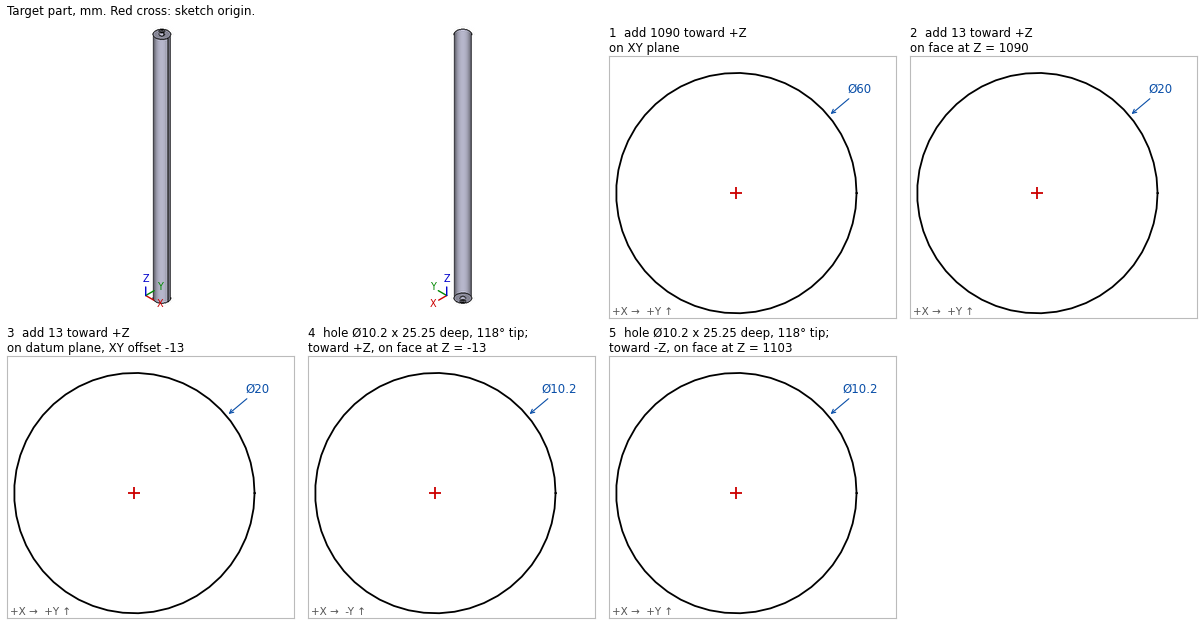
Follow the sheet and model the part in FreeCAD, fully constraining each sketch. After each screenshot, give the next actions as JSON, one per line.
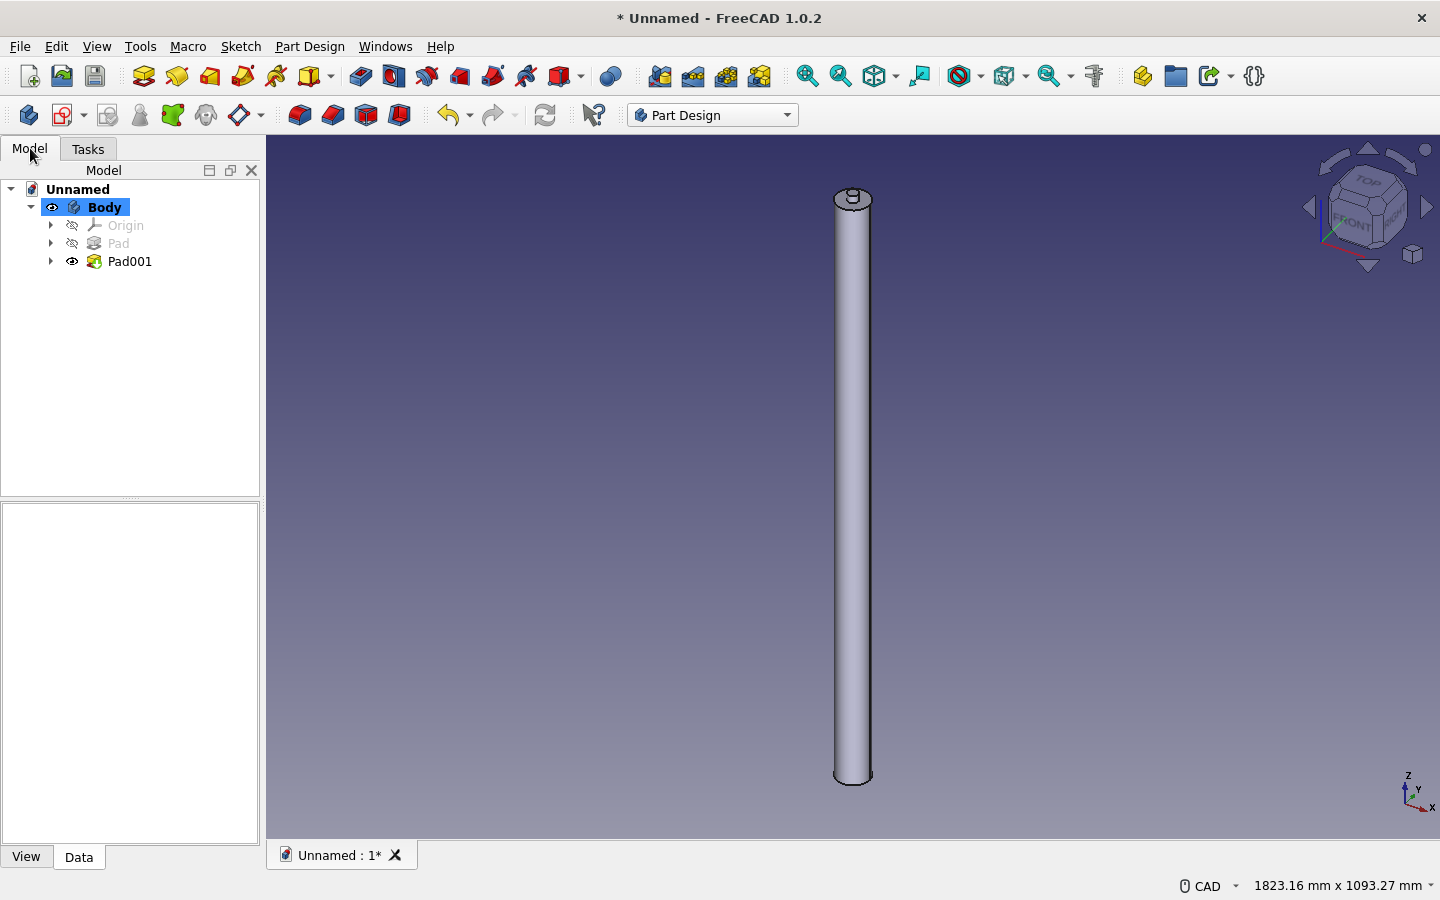
{"action": "left_click", "coordinate": [51, 225]}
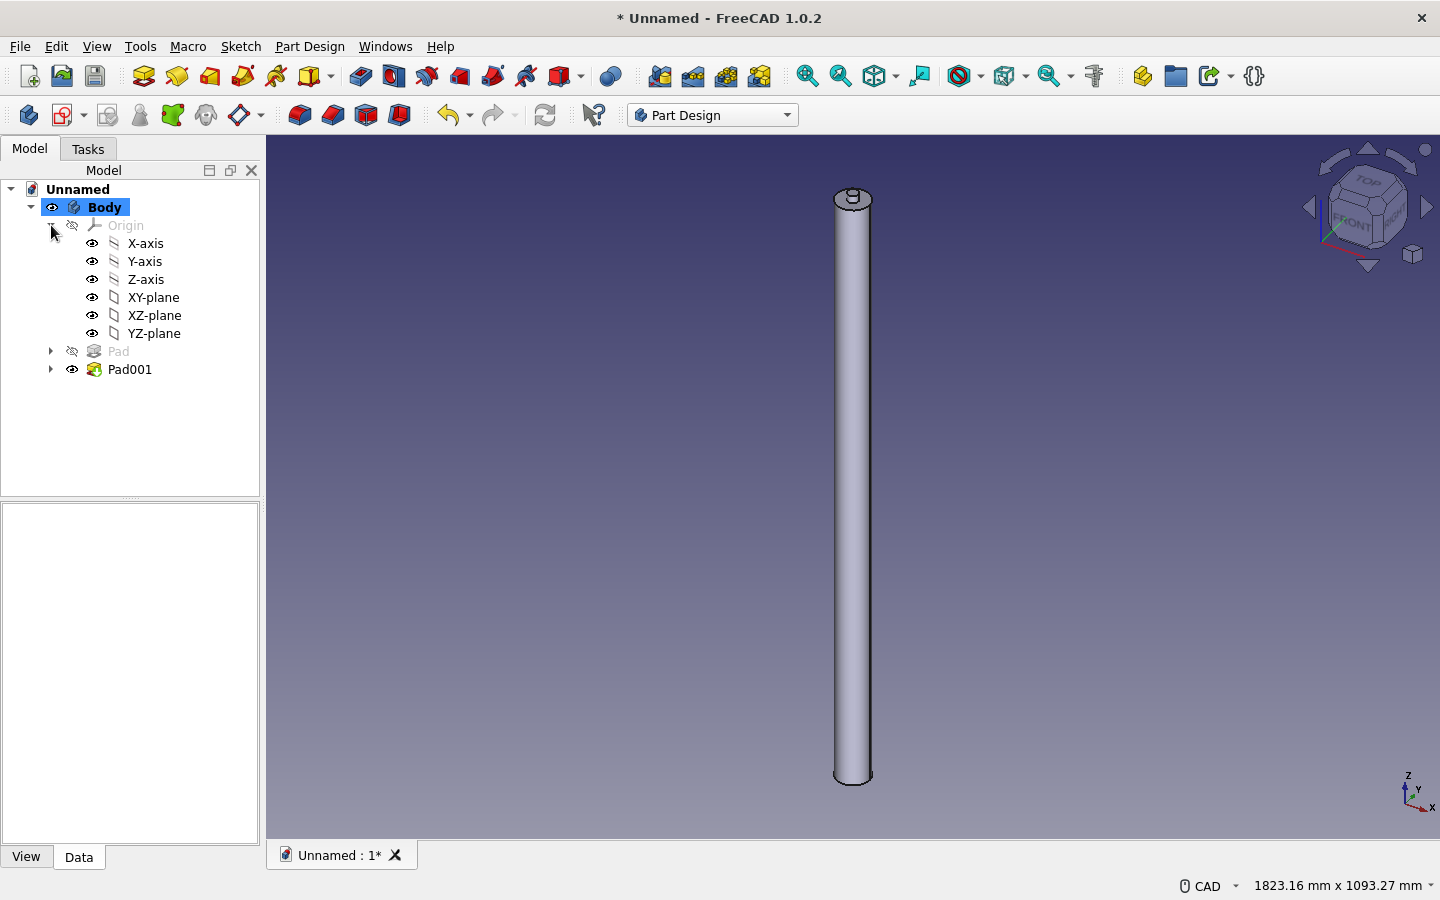
{"action": "left_click", "coordinate": [137, 297]}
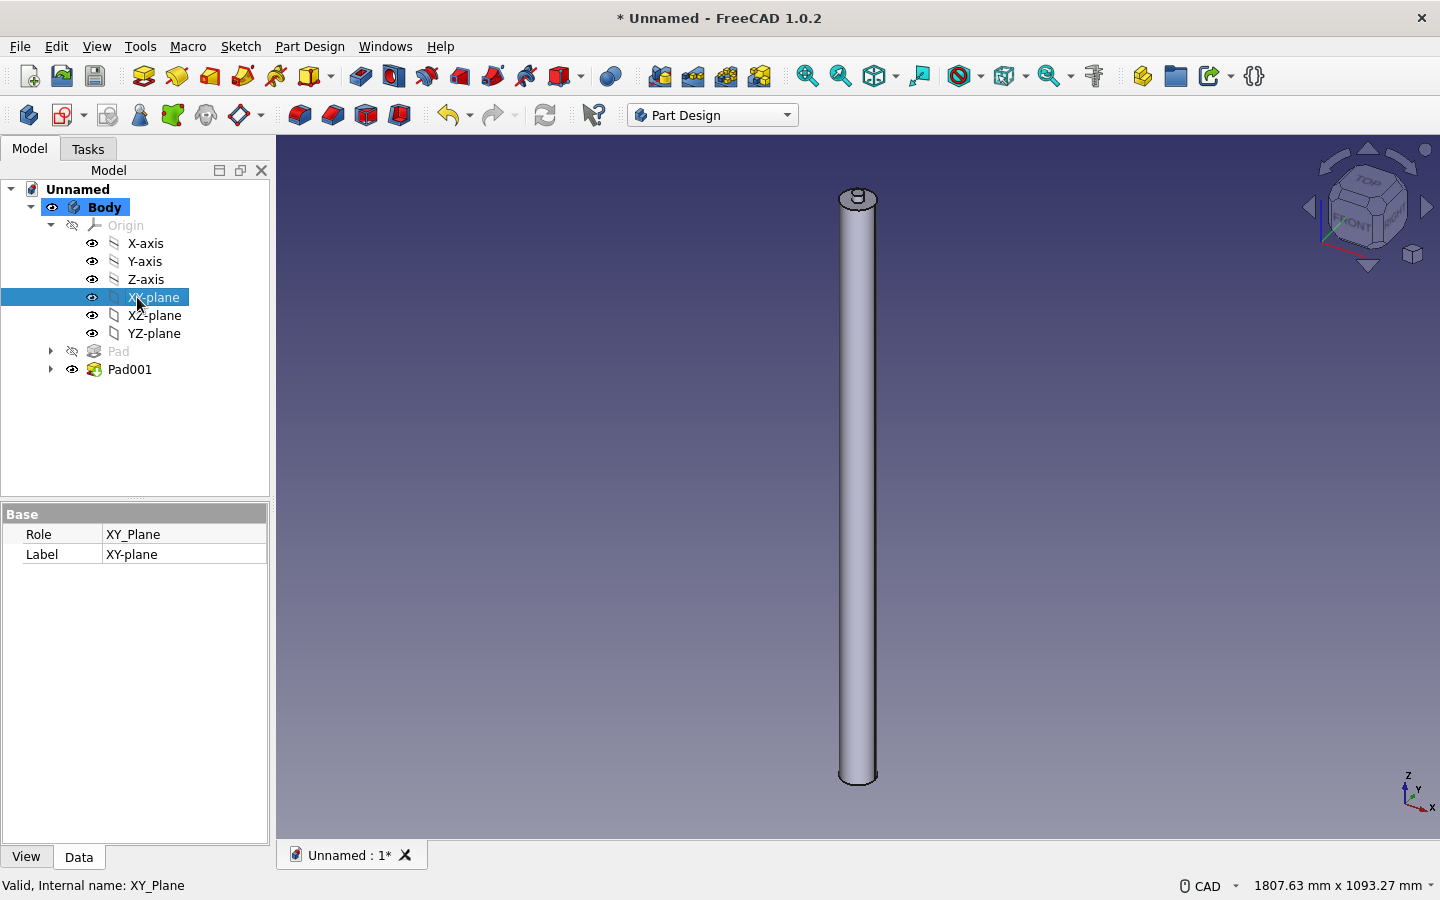
{"action": "left_click", "coordinate": [238, 116]}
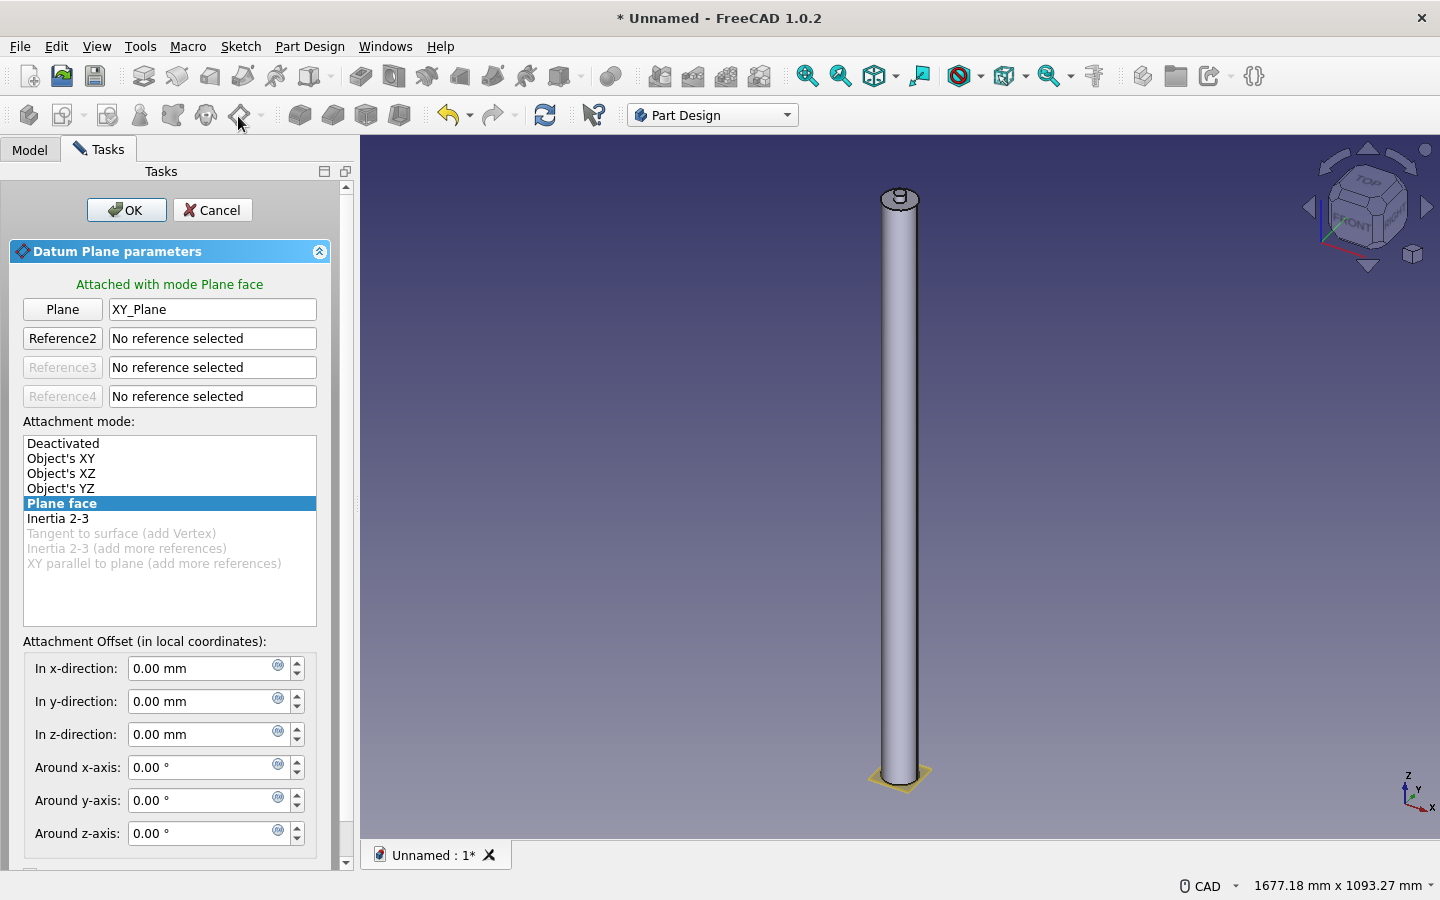
{"action": "triple_click", "coordinate": [210, 734]}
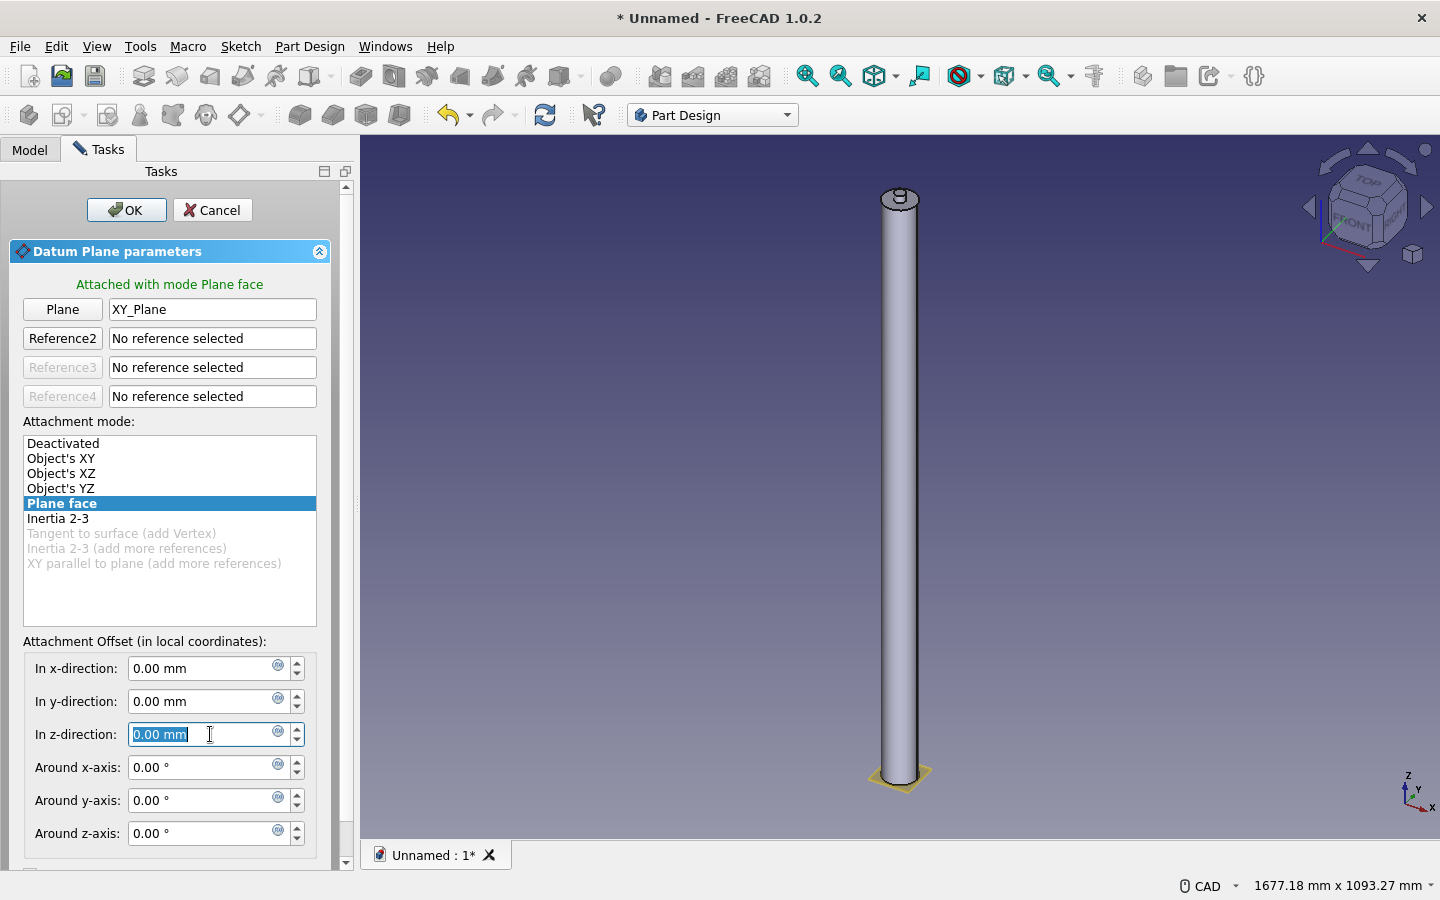
{"action": "type", "text": "-13"}
{"action": "key", "text": "Tab"}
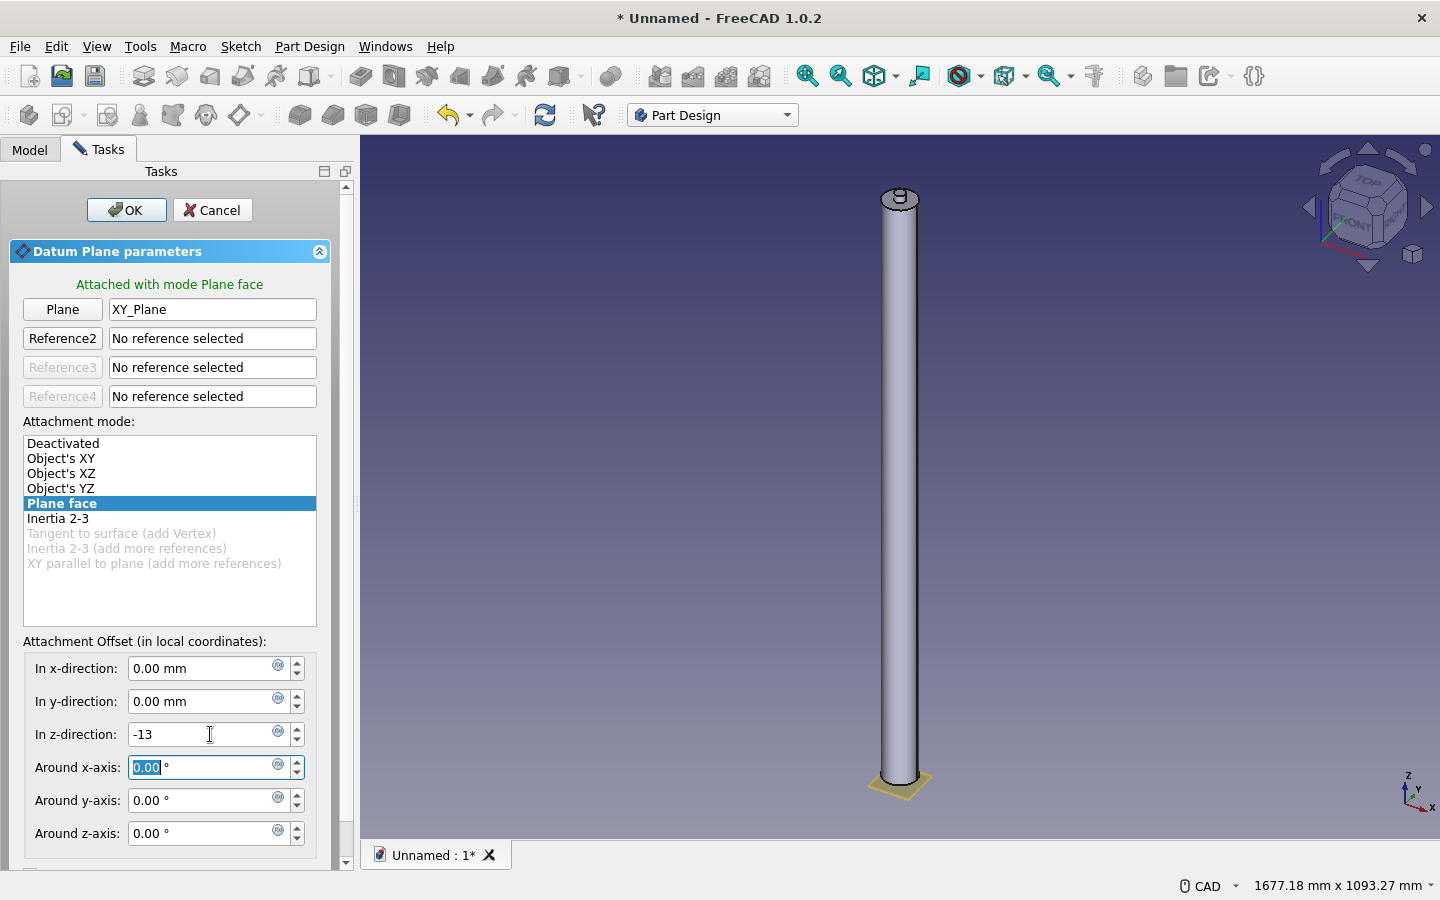
{"action": "left_click", "coordinate": [127, 210]}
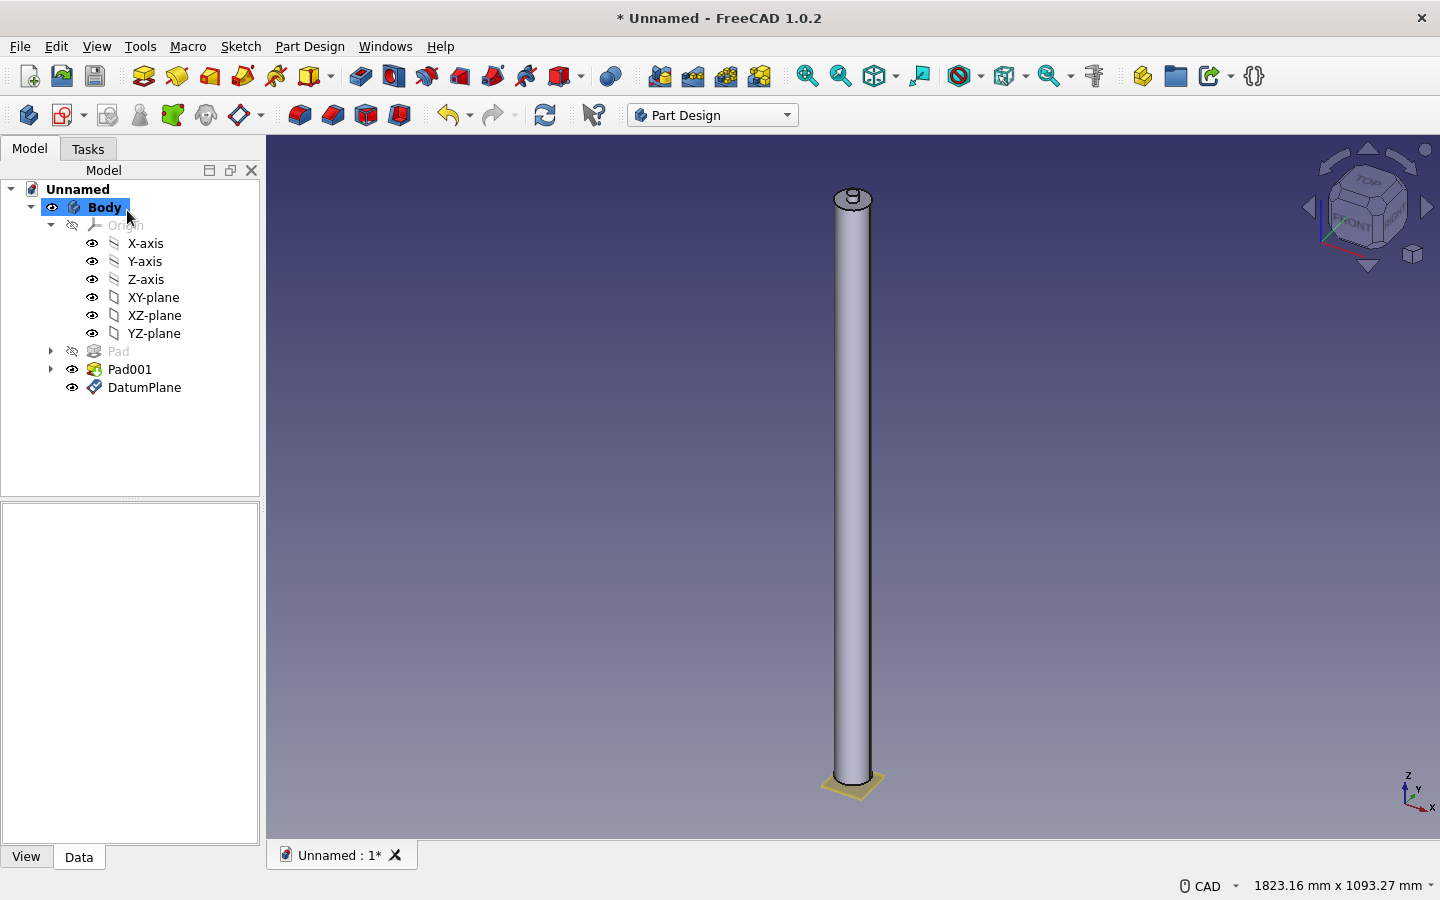
{"action": "left_click", "coordinate": [117, 387]}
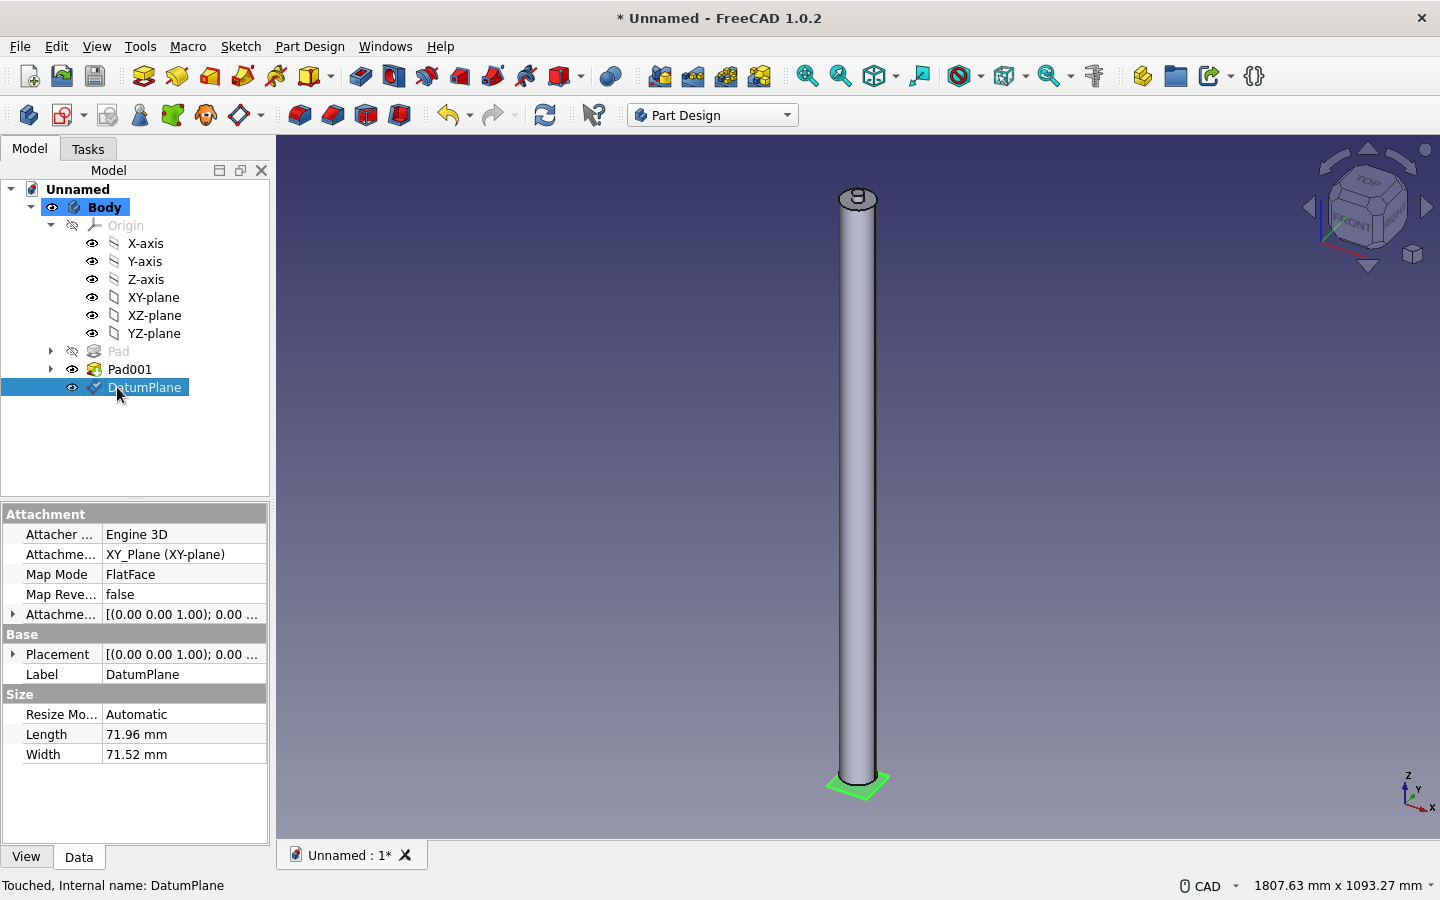
{"action": "left_click", "coordinate": [62, 116]}